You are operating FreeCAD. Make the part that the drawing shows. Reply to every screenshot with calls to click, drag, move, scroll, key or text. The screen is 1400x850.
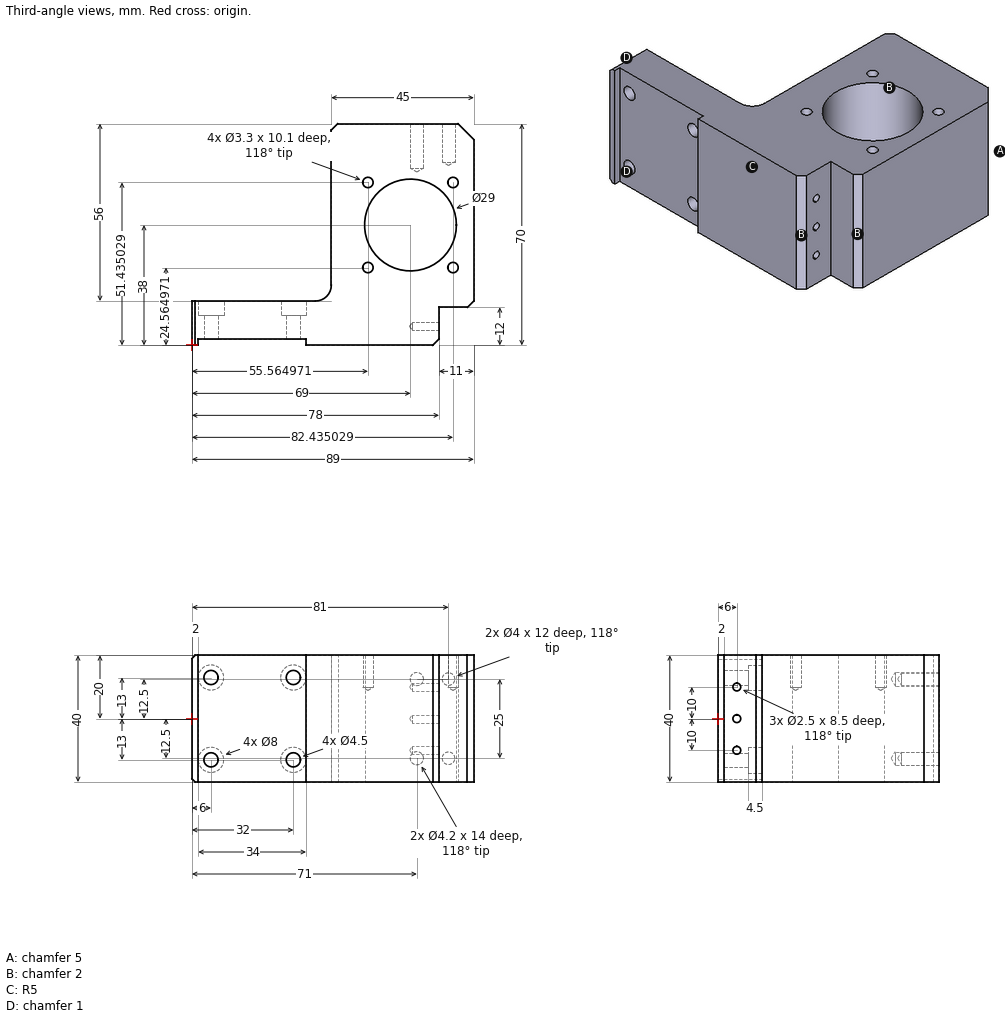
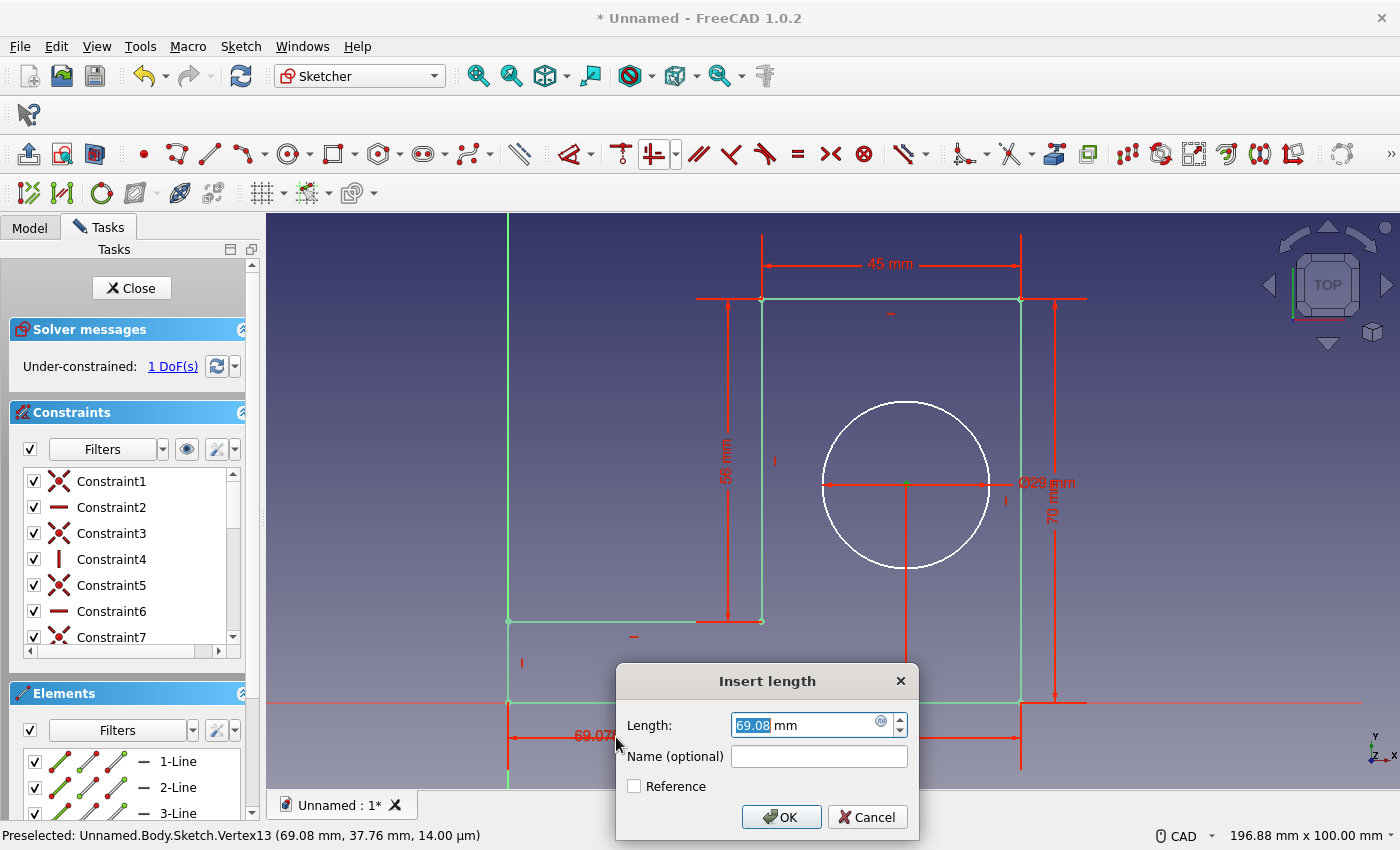
text(69)
key(Return)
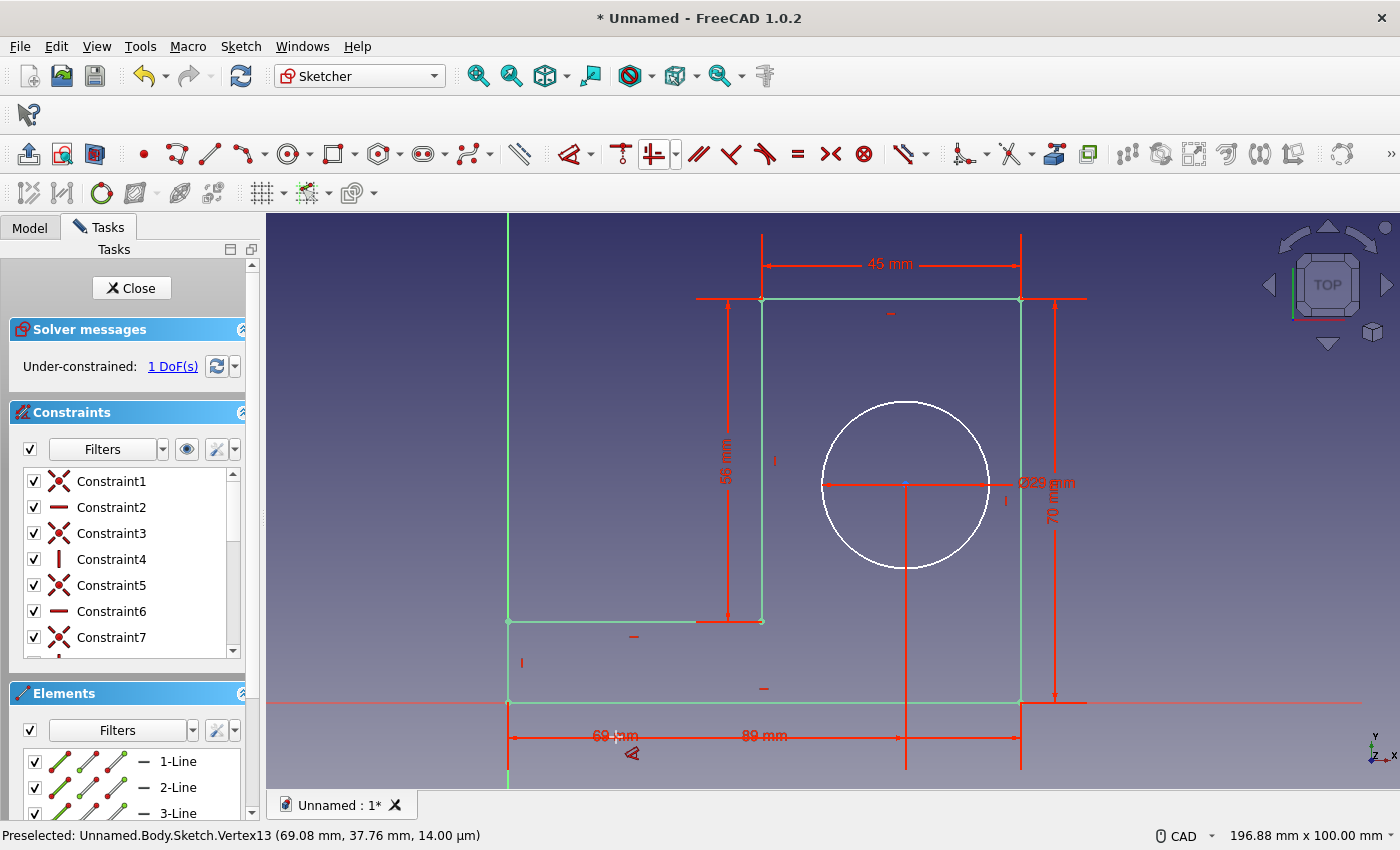
click(906, 485)
click(474, 594)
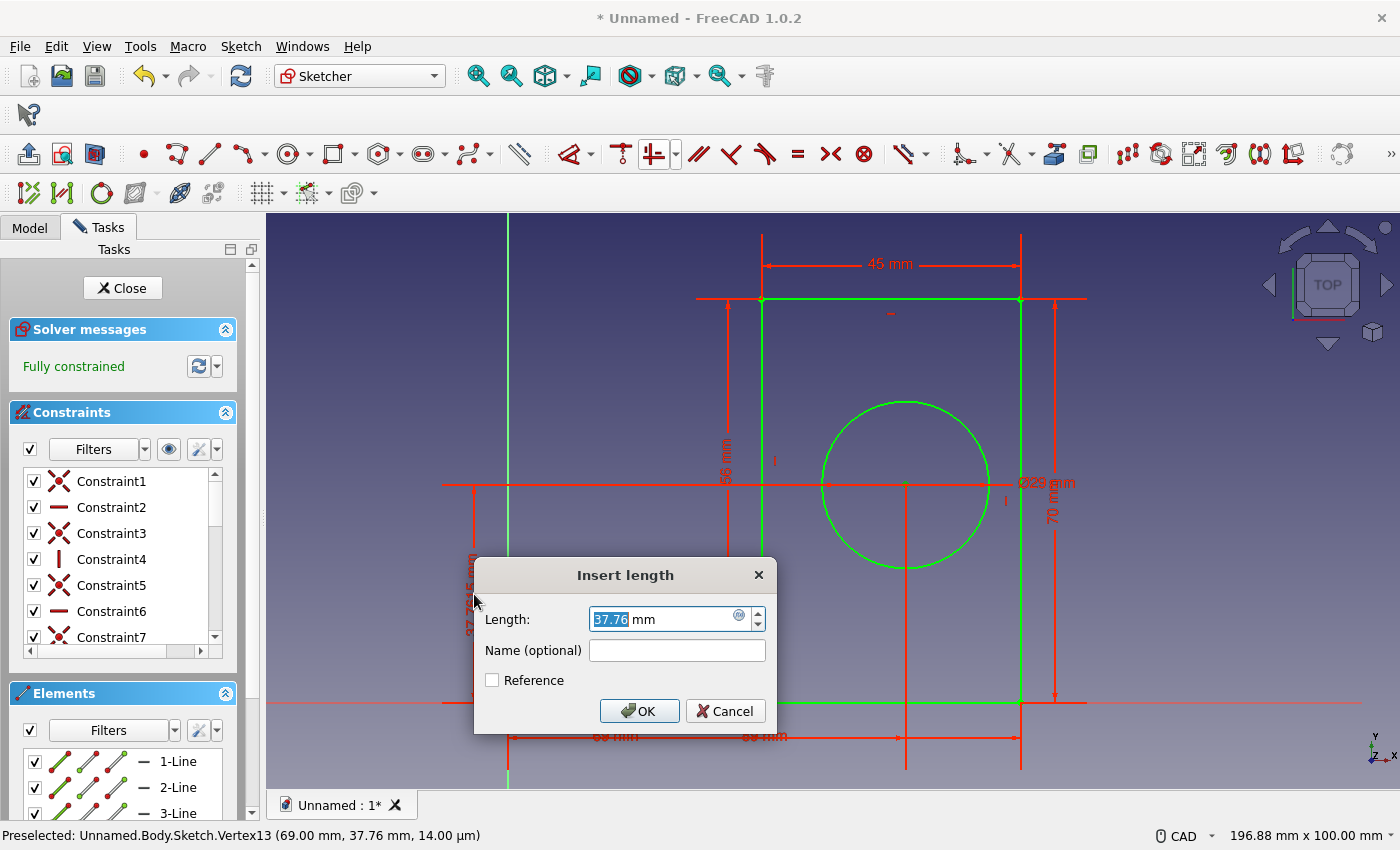
text(38)
key(Return)
key(Escape)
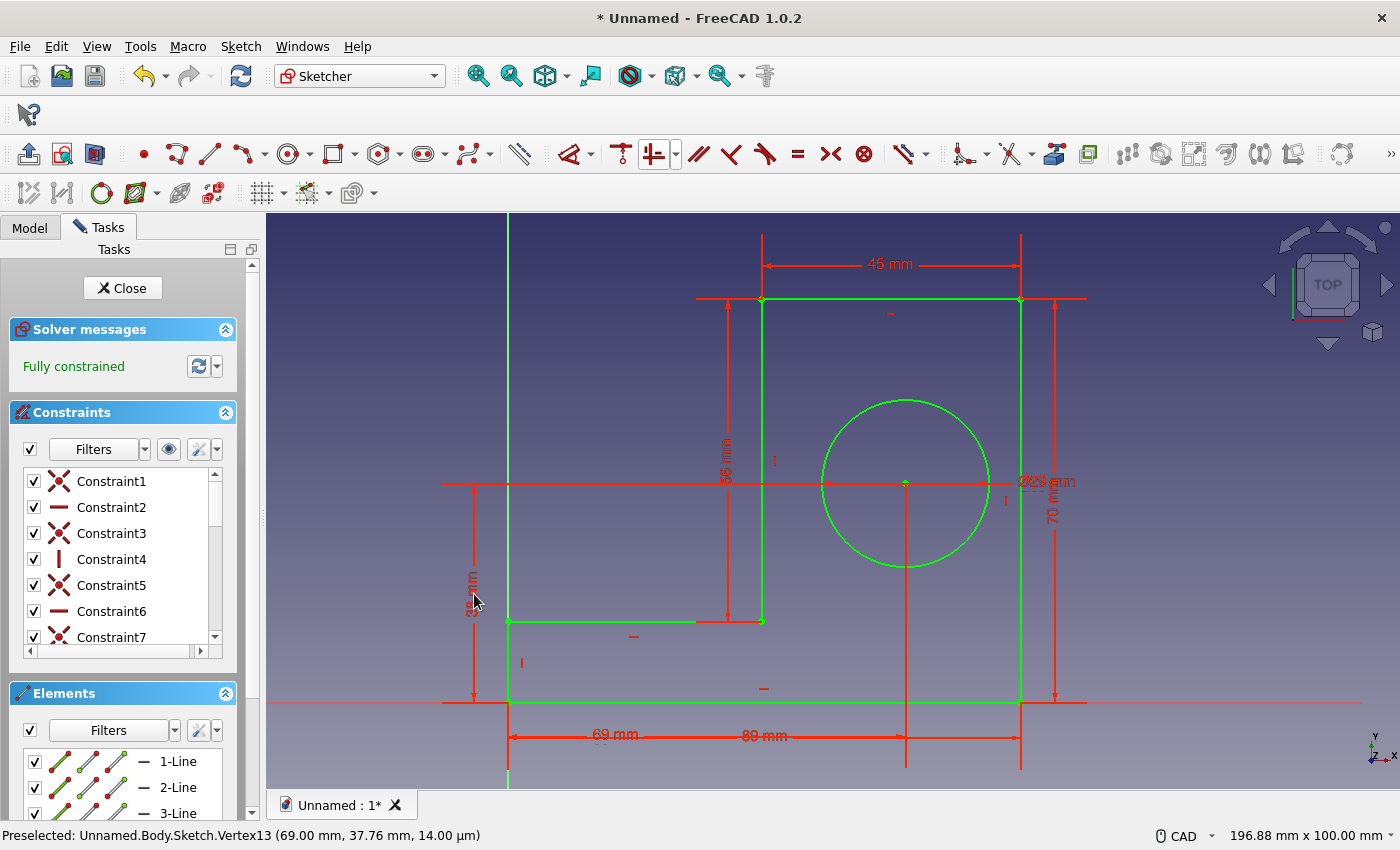
click(123, 288)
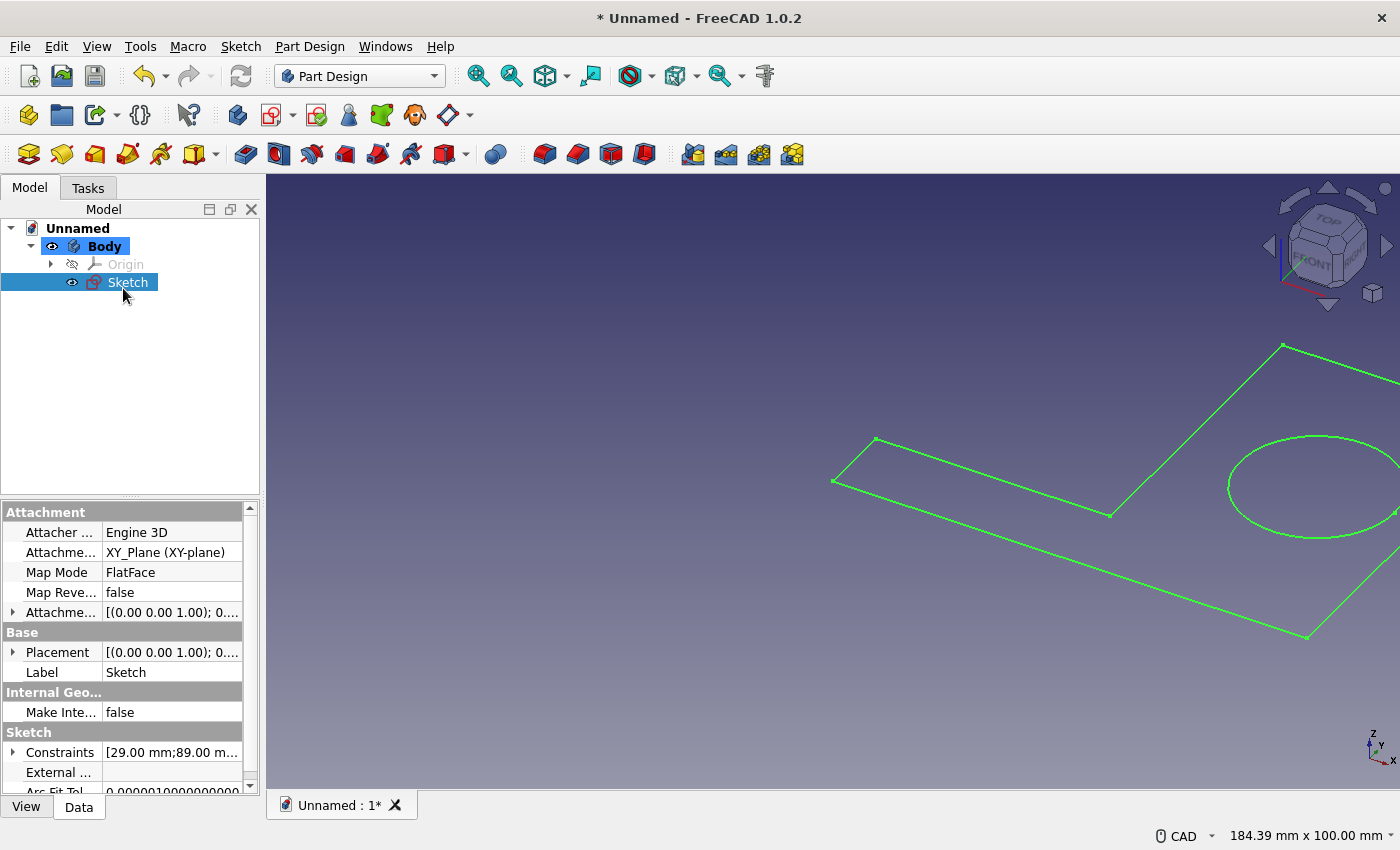
click(29, 154)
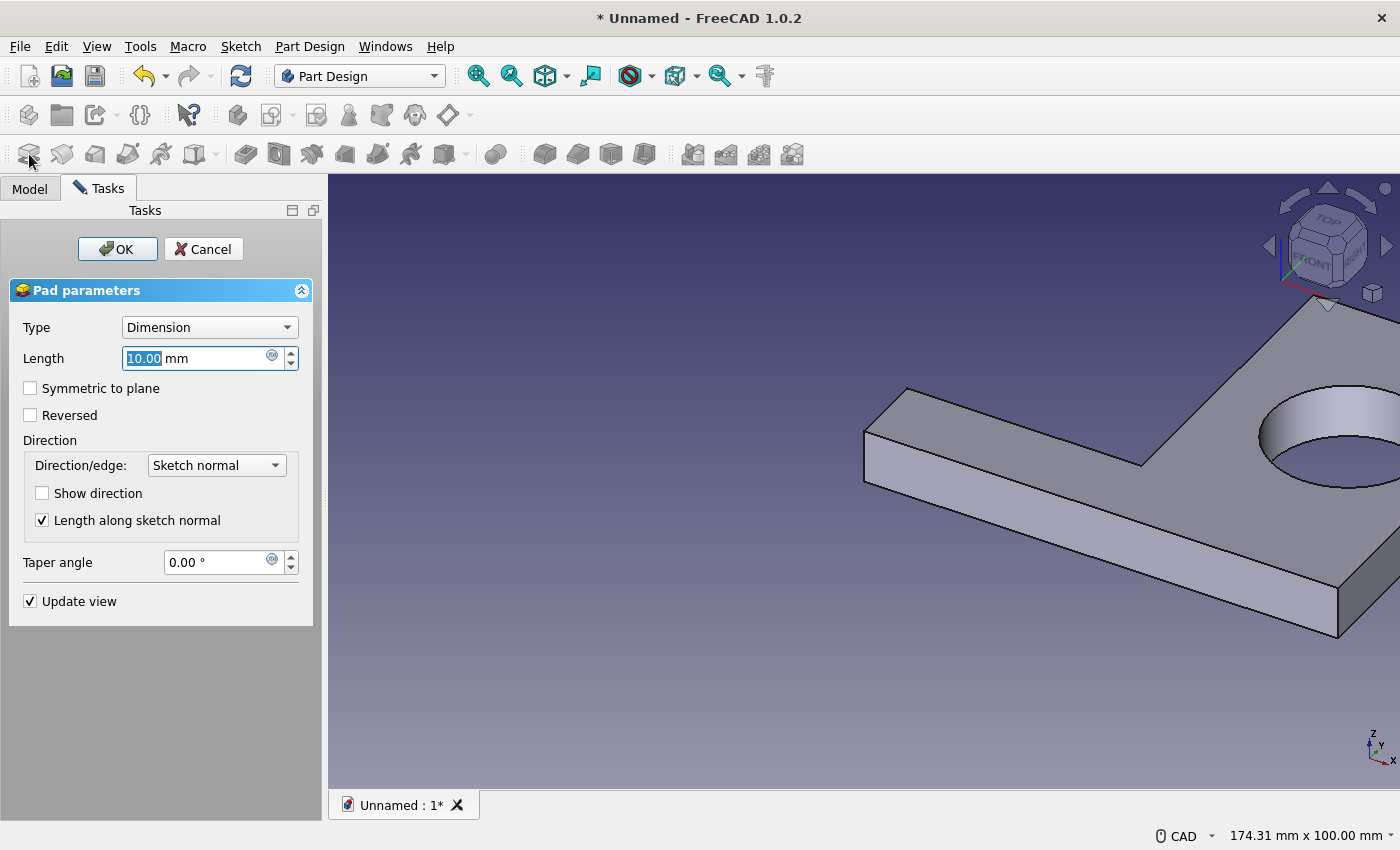
text(40)
key(Tab)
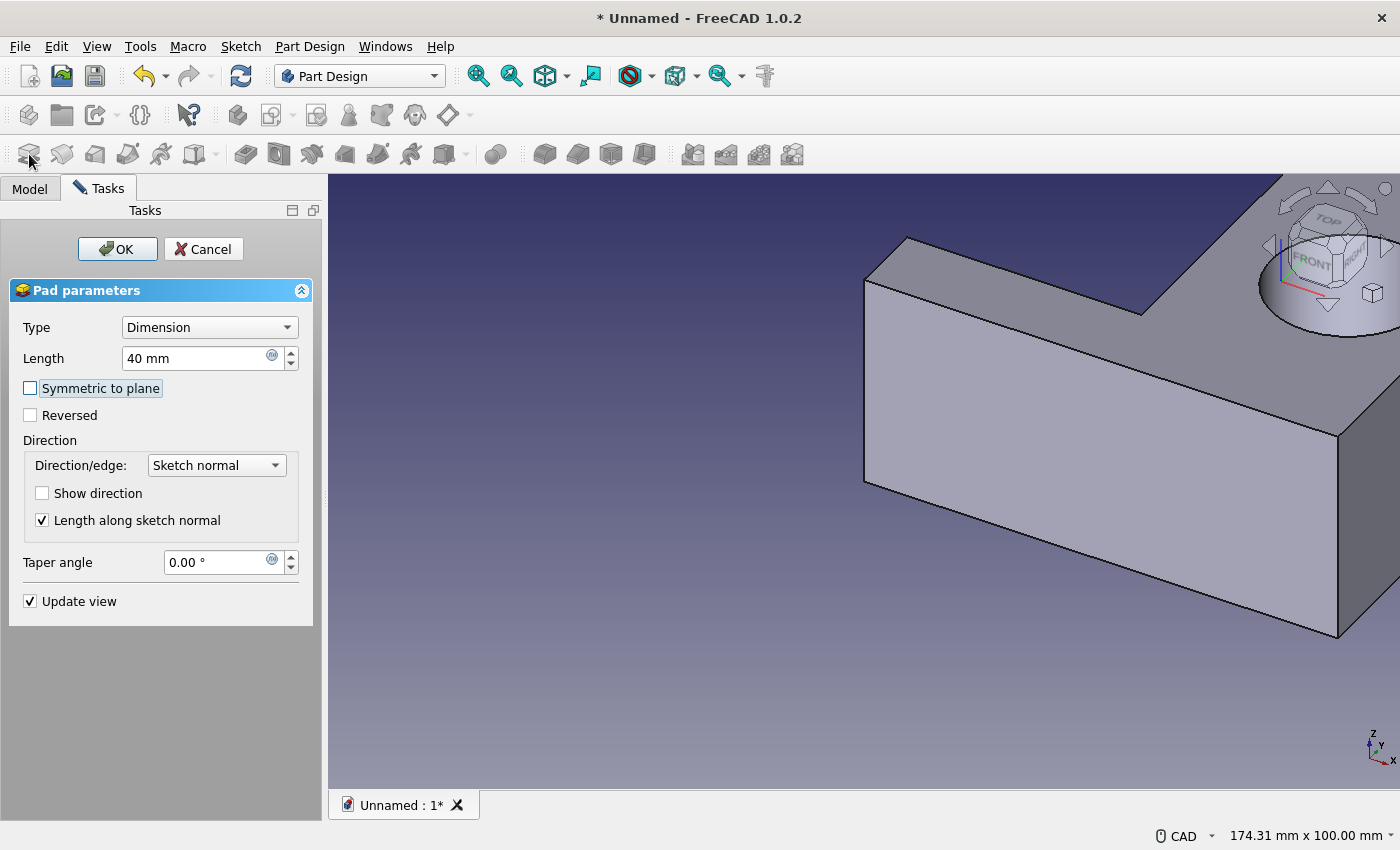
click(31, 388)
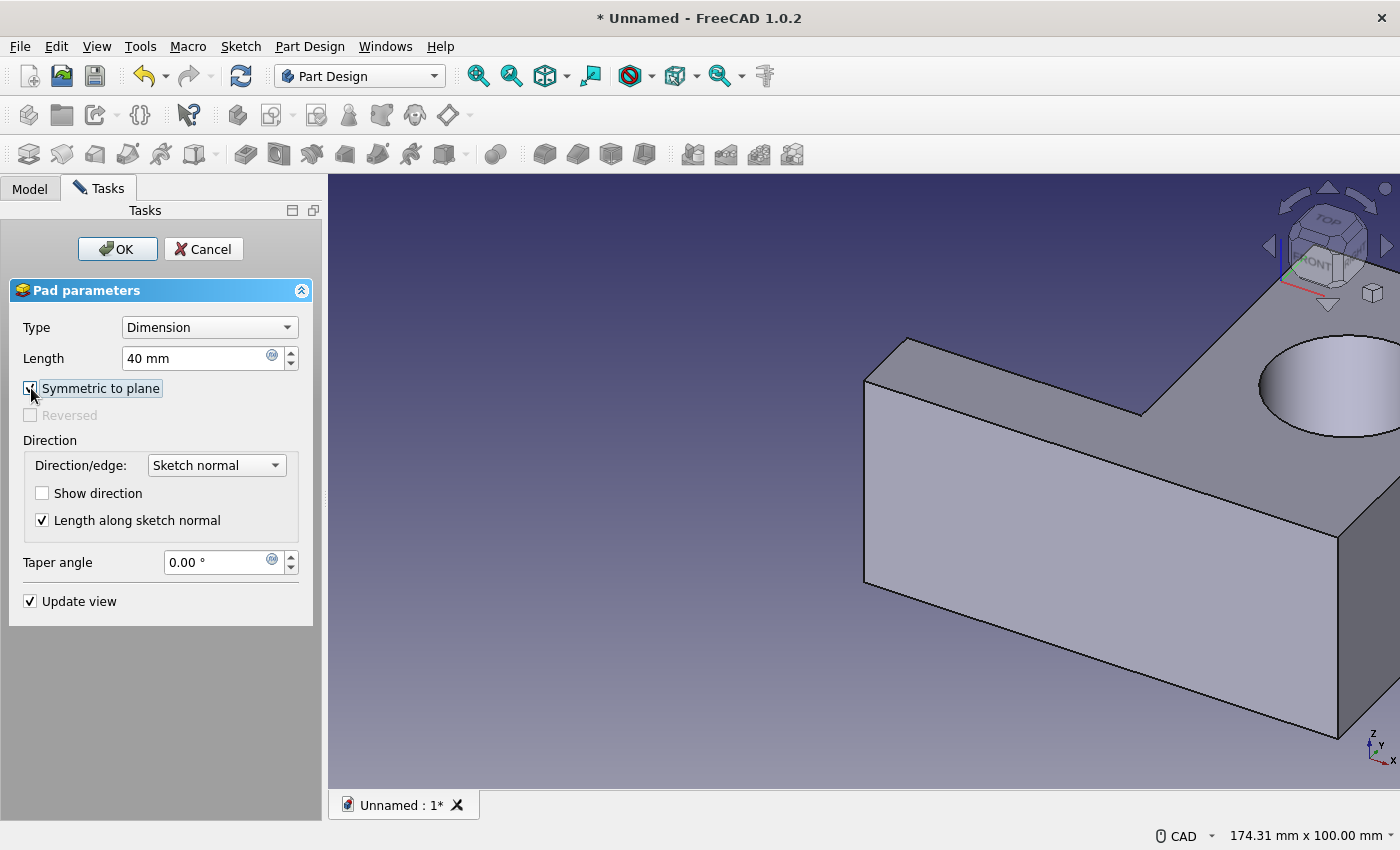
click(118, 249)